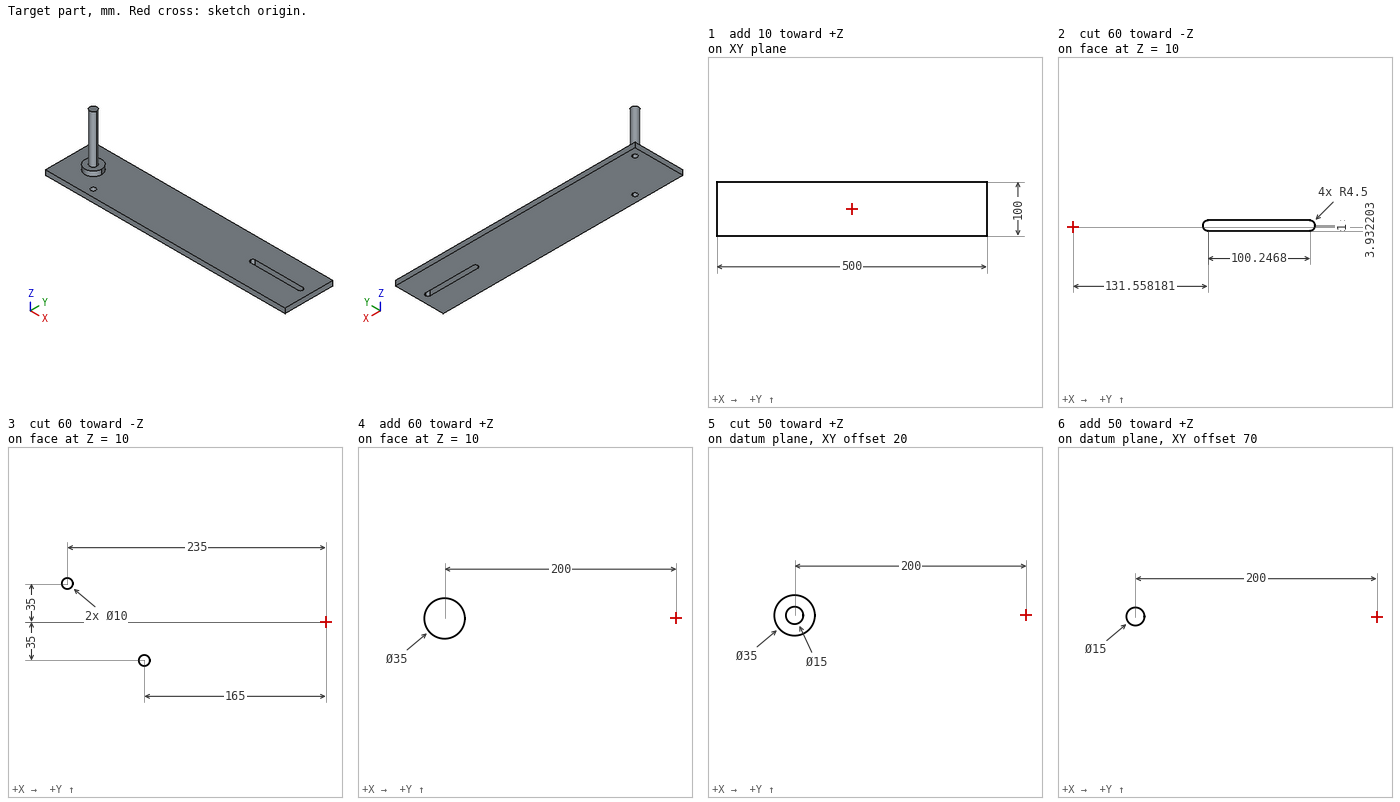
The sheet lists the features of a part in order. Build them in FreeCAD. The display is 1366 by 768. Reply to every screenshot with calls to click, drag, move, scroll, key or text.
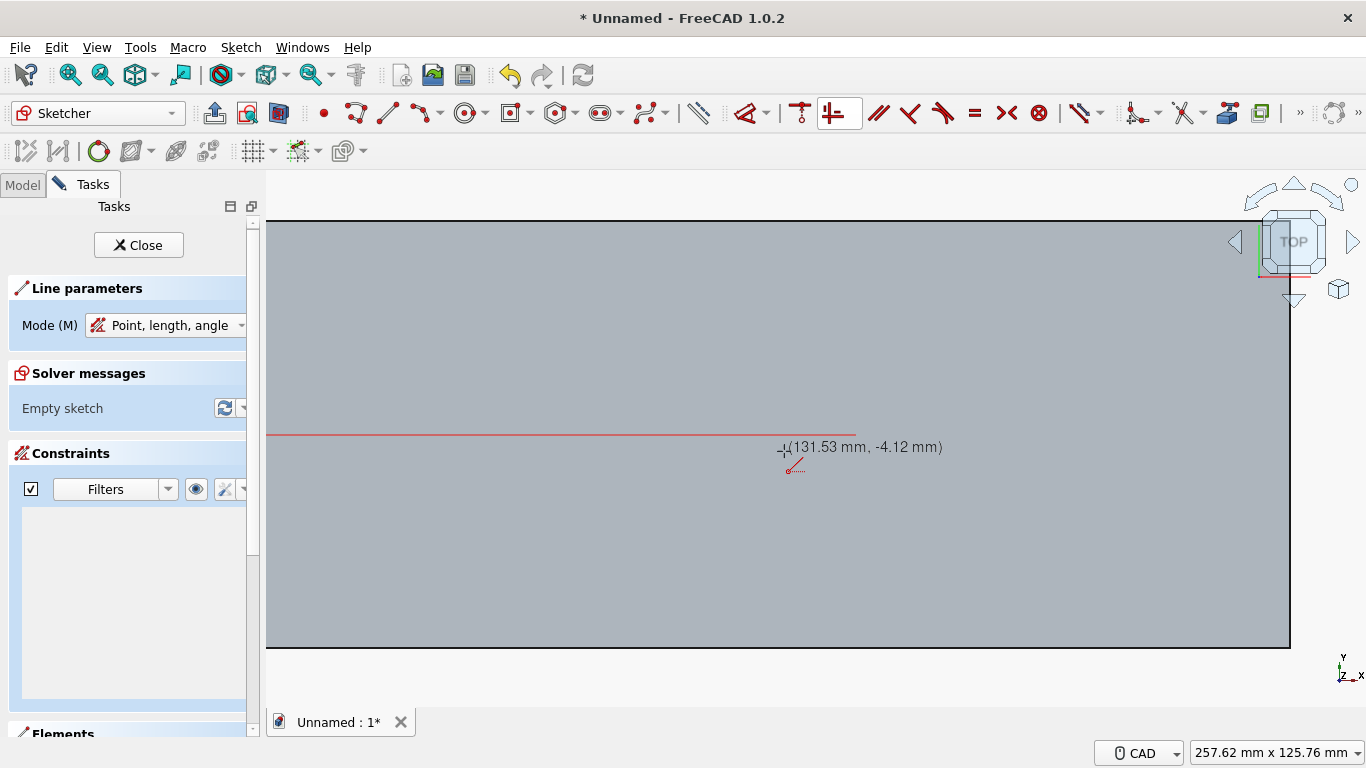
click(784, 451)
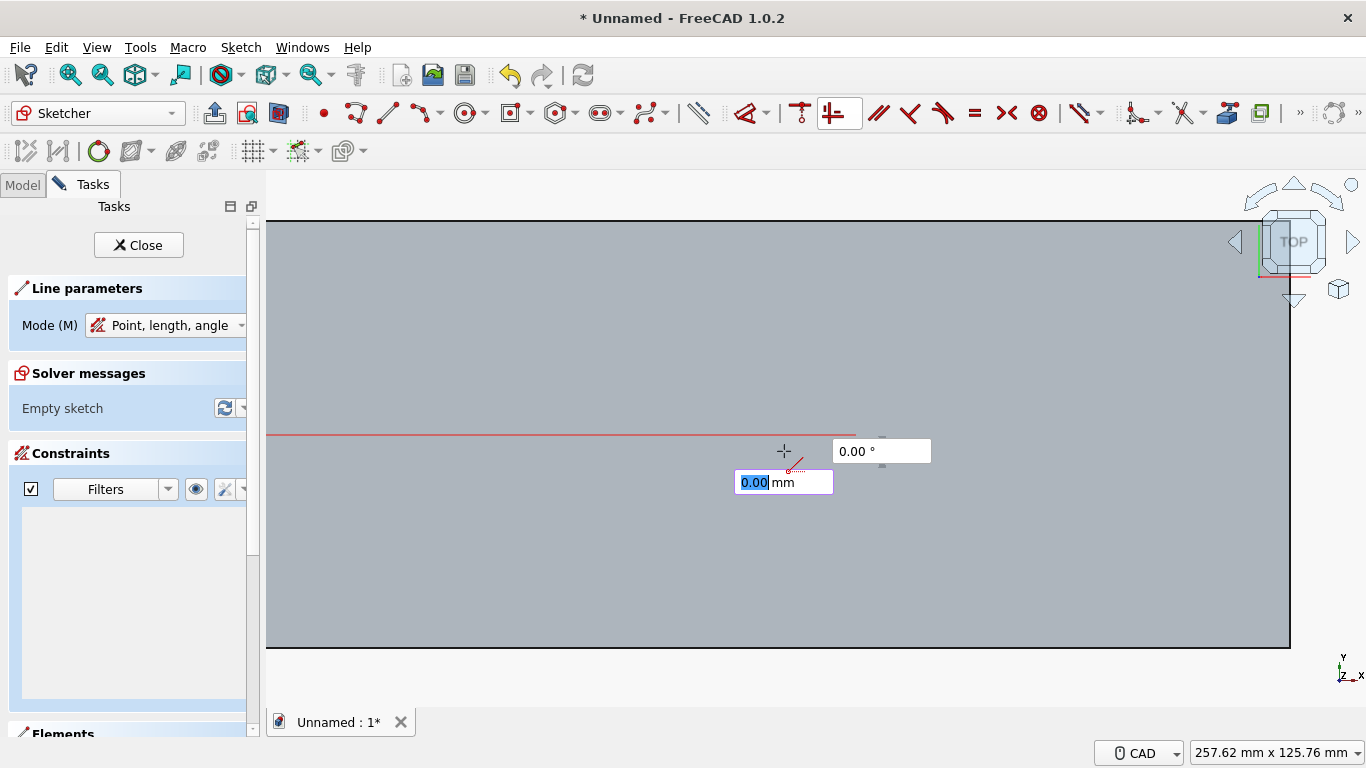
scroll(790, 456, down, 2)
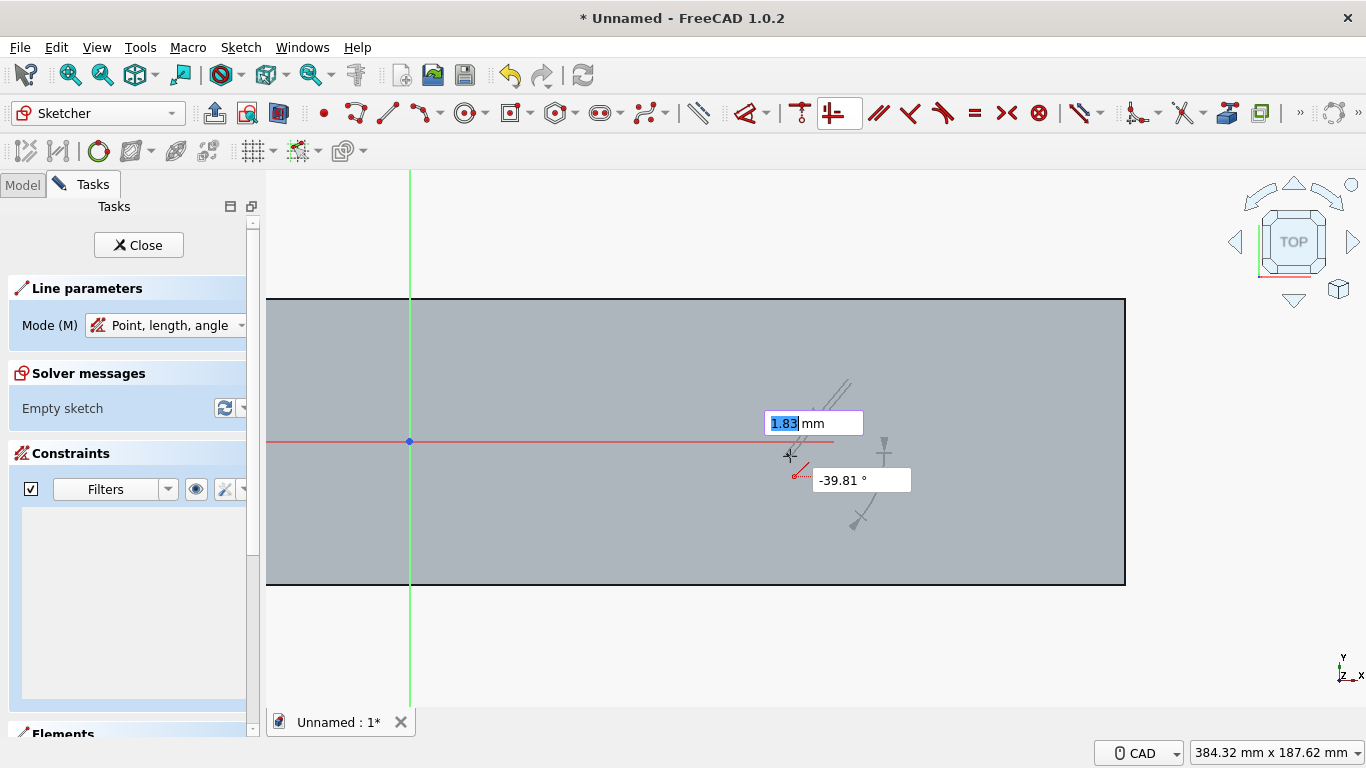
scroll(1073, 453, up, 2)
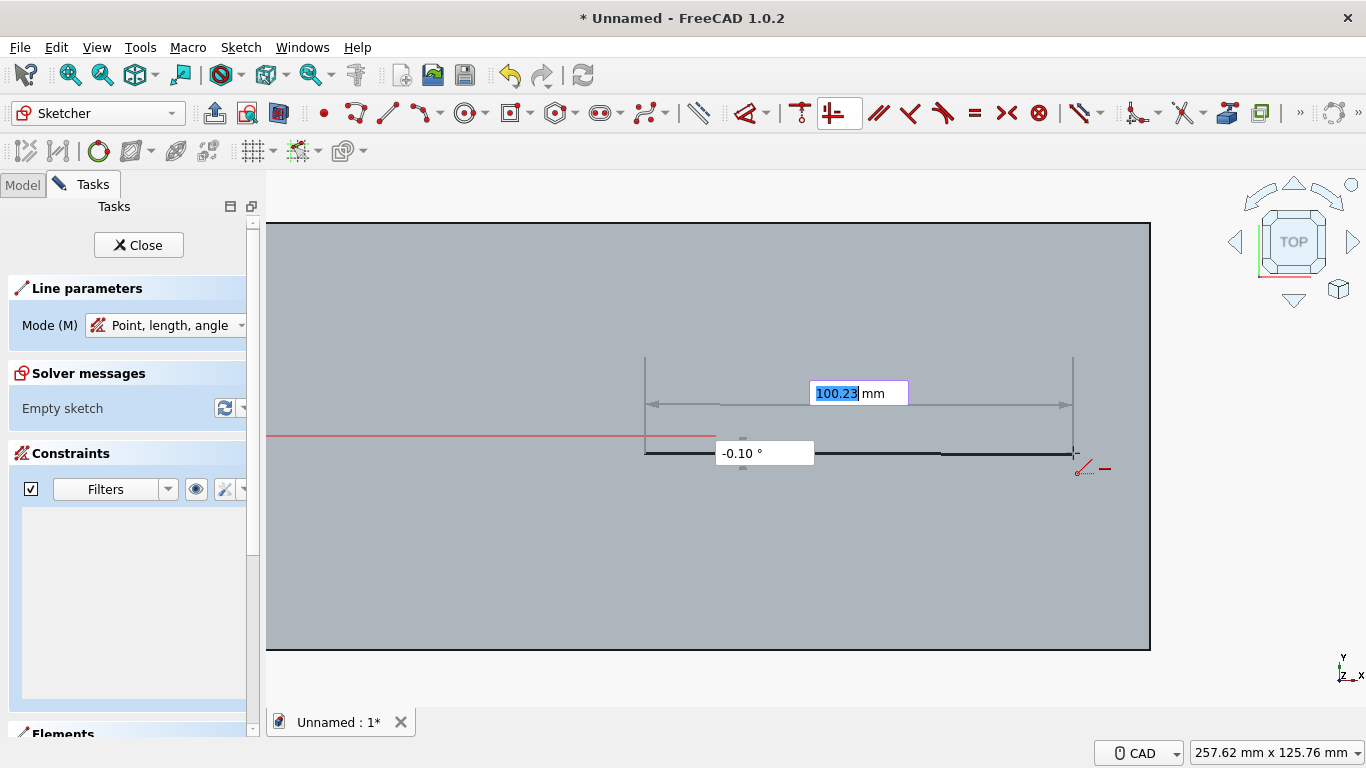
click(1073, 452)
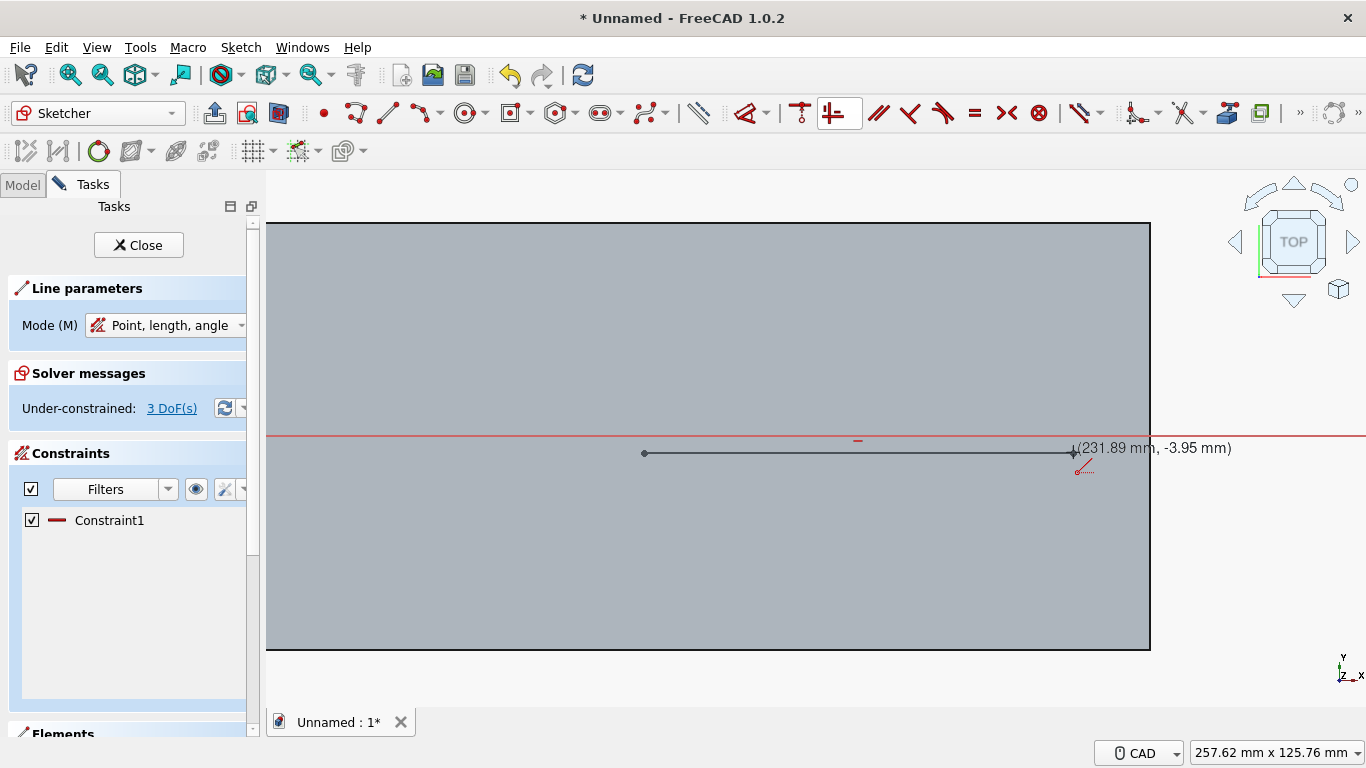
scroll(1092, 434, up, 10)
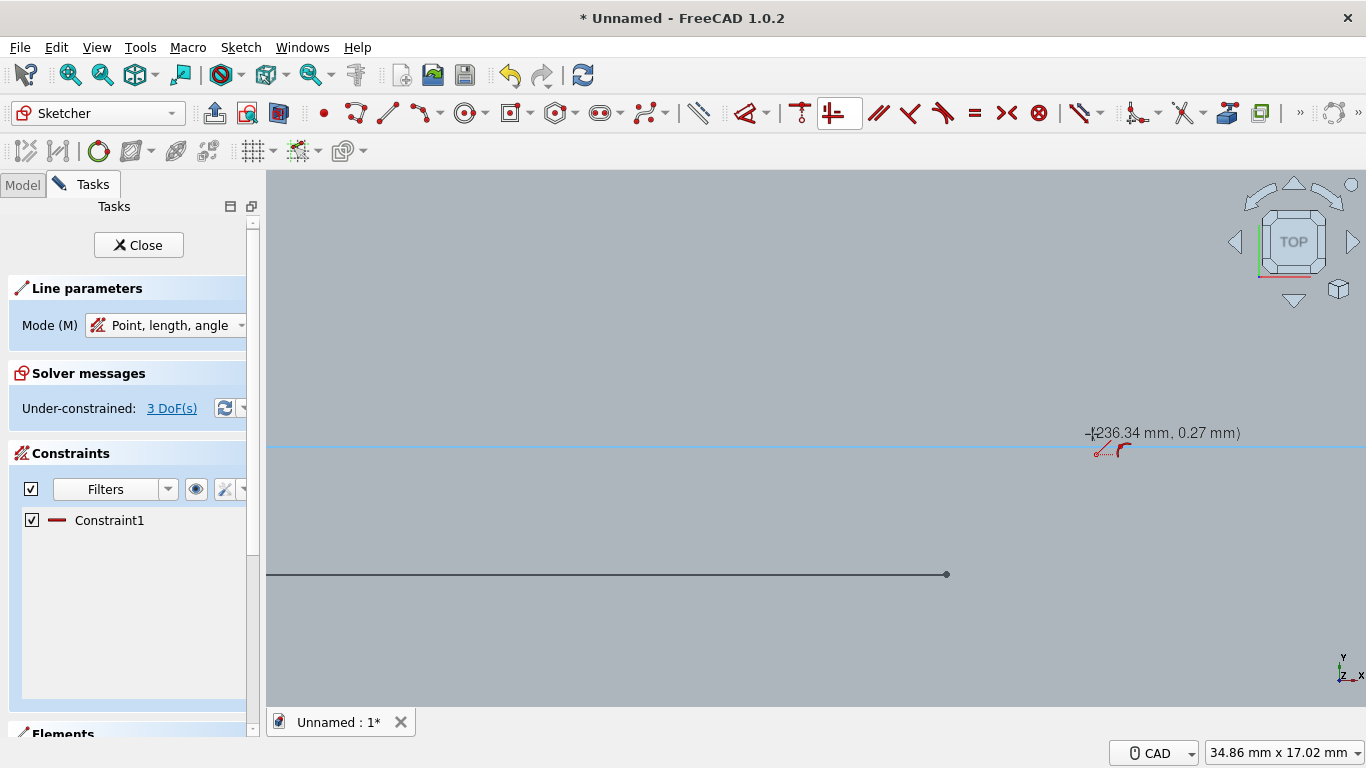
click(1086, 429)
click(1086, 397)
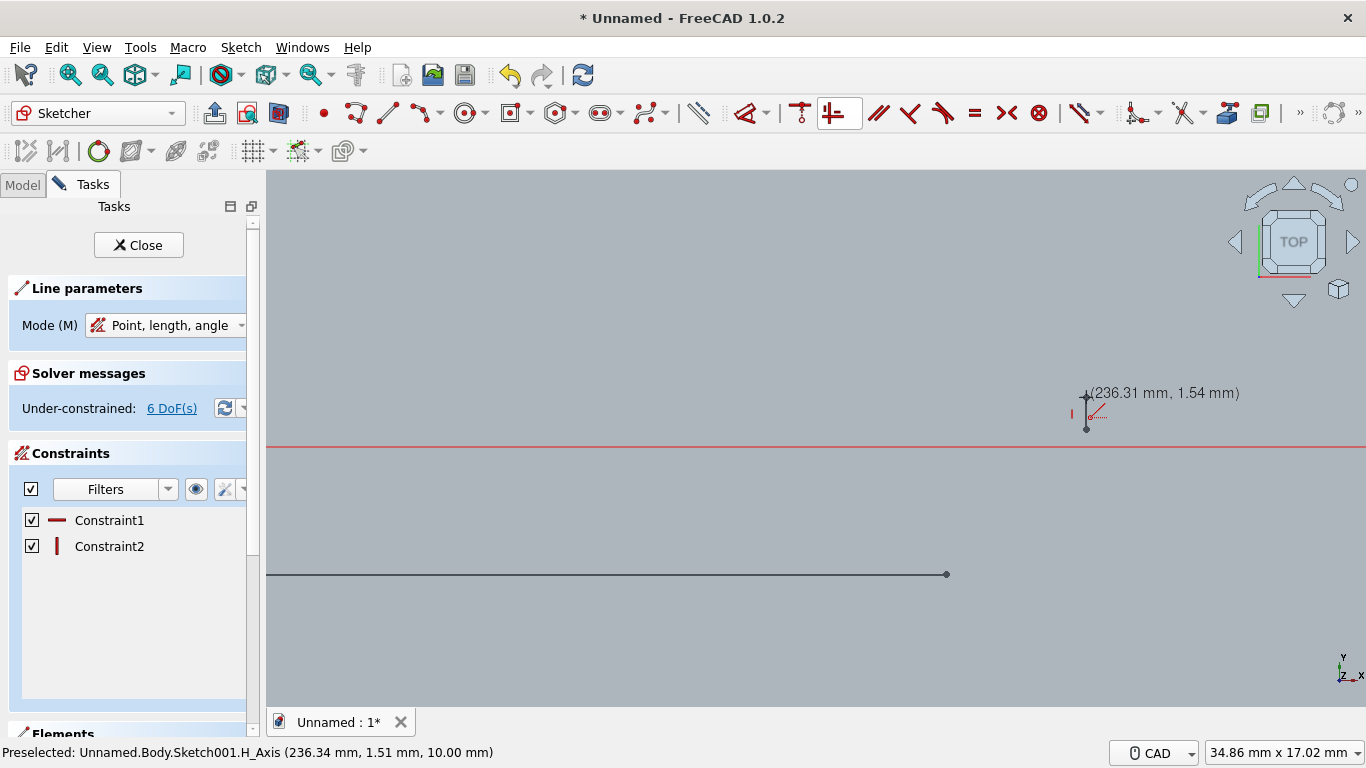
scroll(1086, 441, down, 12)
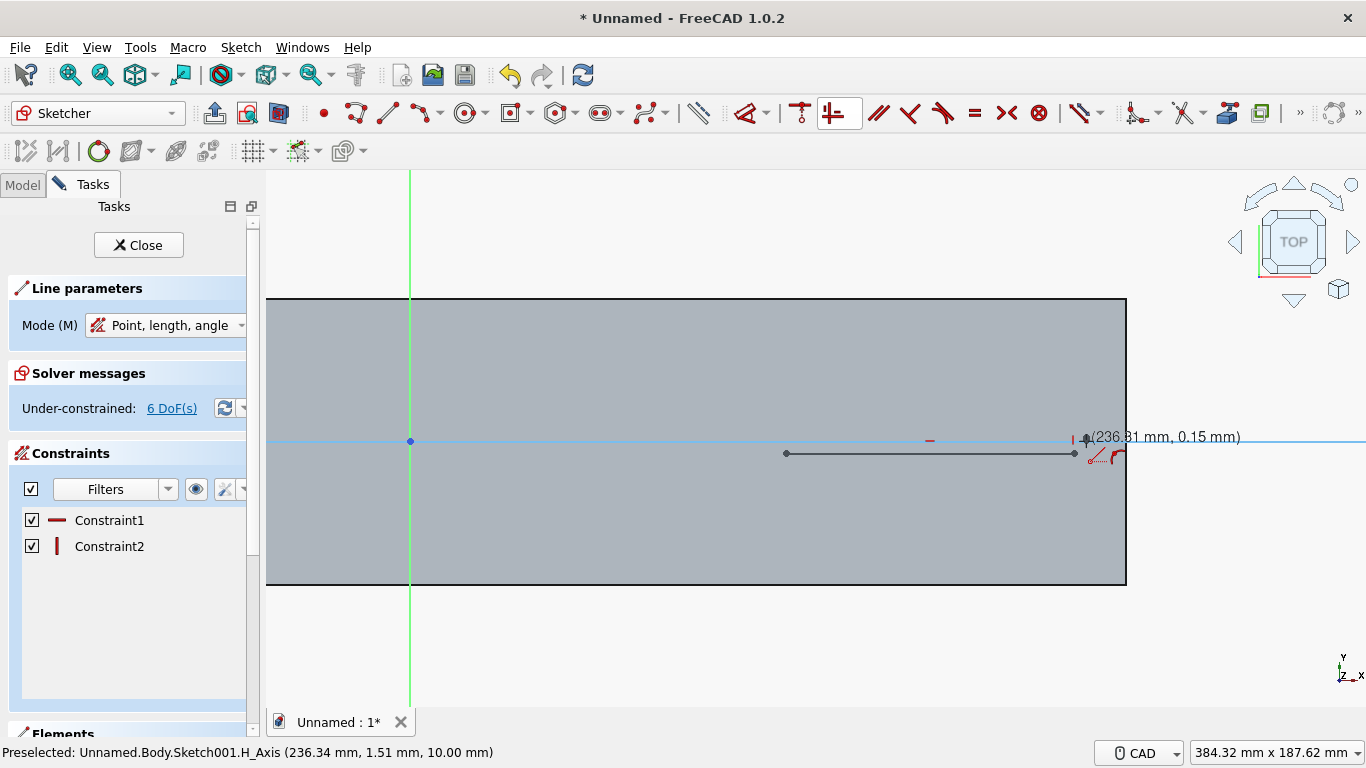
click(1074, 425)
click(787, 425)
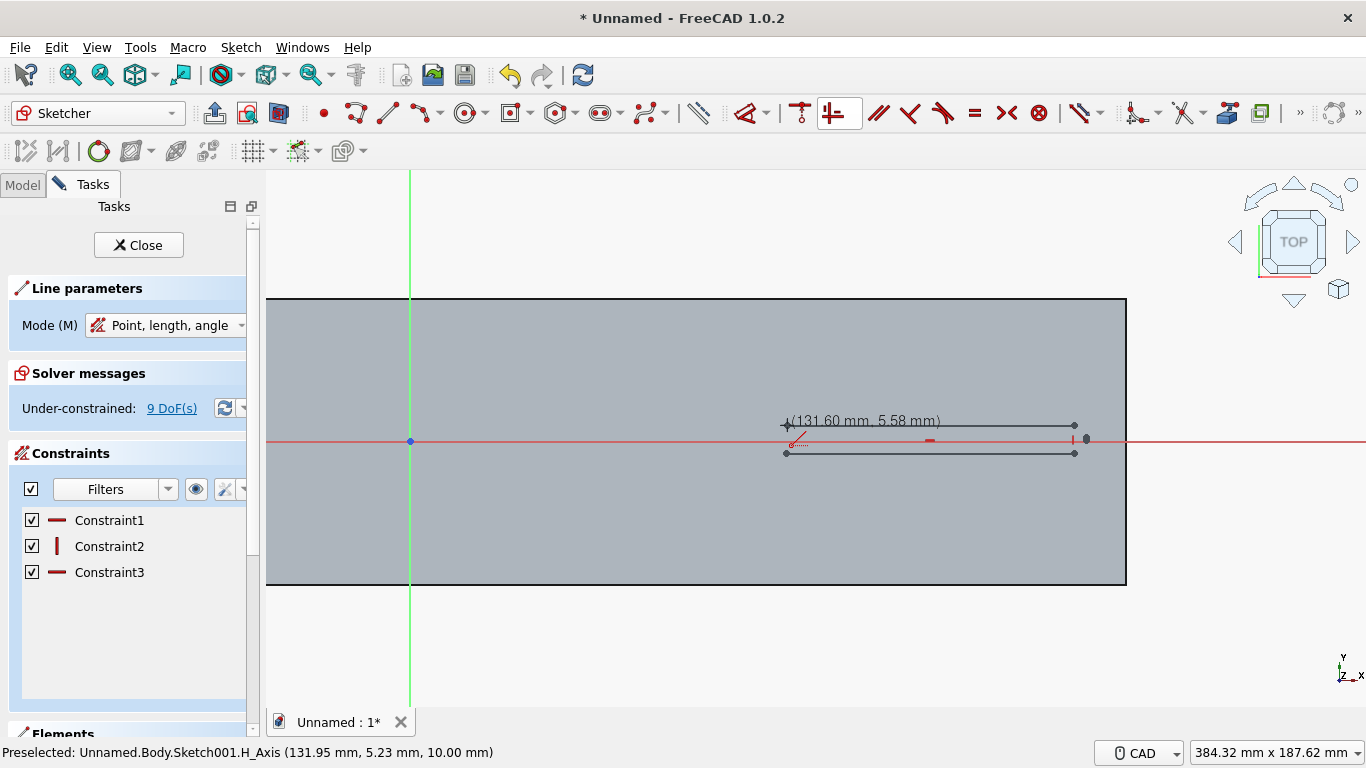
scroll(774, 437, up, 7)